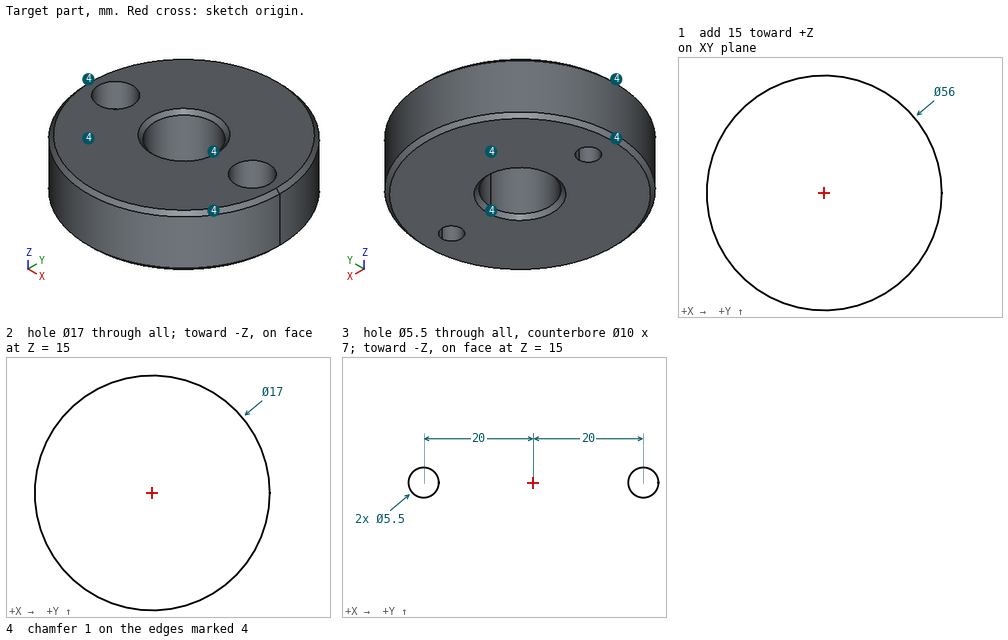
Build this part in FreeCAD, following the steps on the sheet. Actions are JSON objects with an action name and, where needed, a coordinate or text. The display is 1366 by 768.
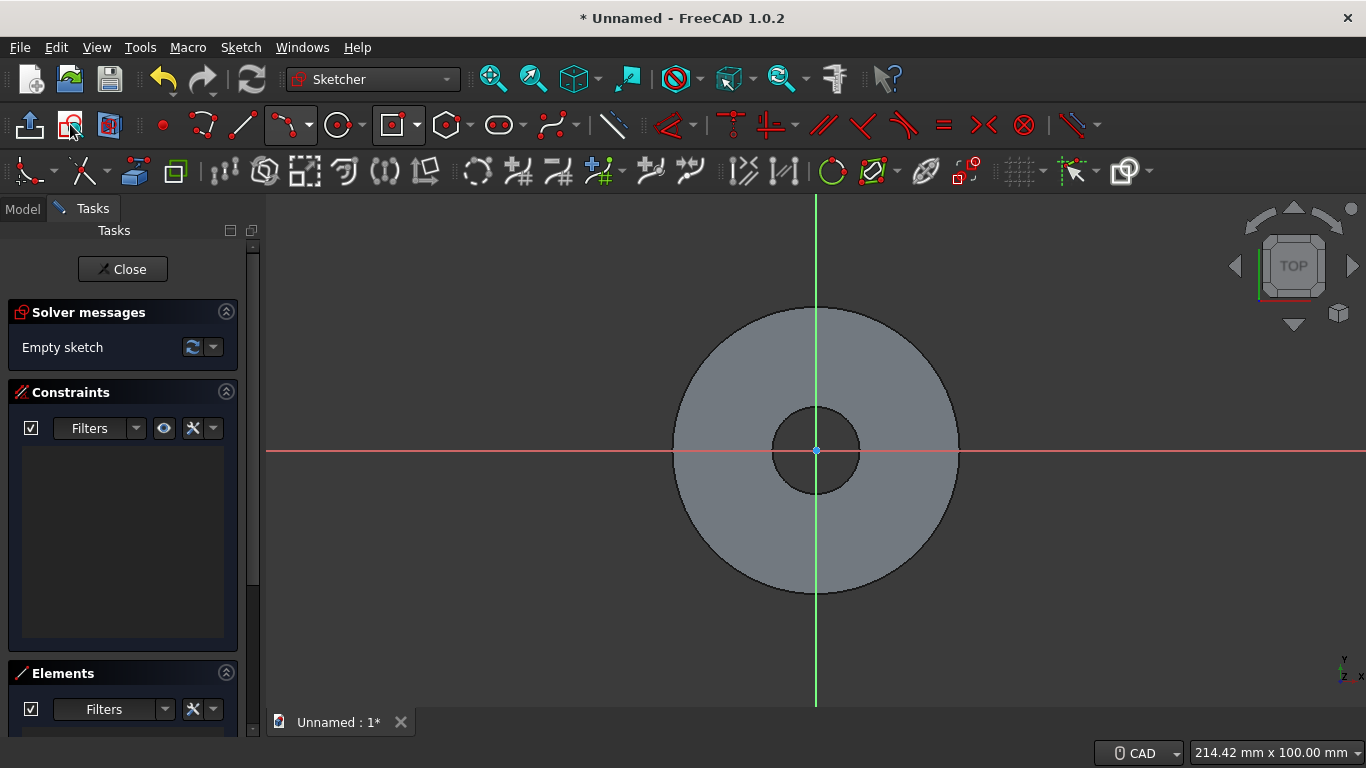
{"action": "scroll", "coordinate": [856, 450], "scroll_direction": "up", "scroll_amount": 5}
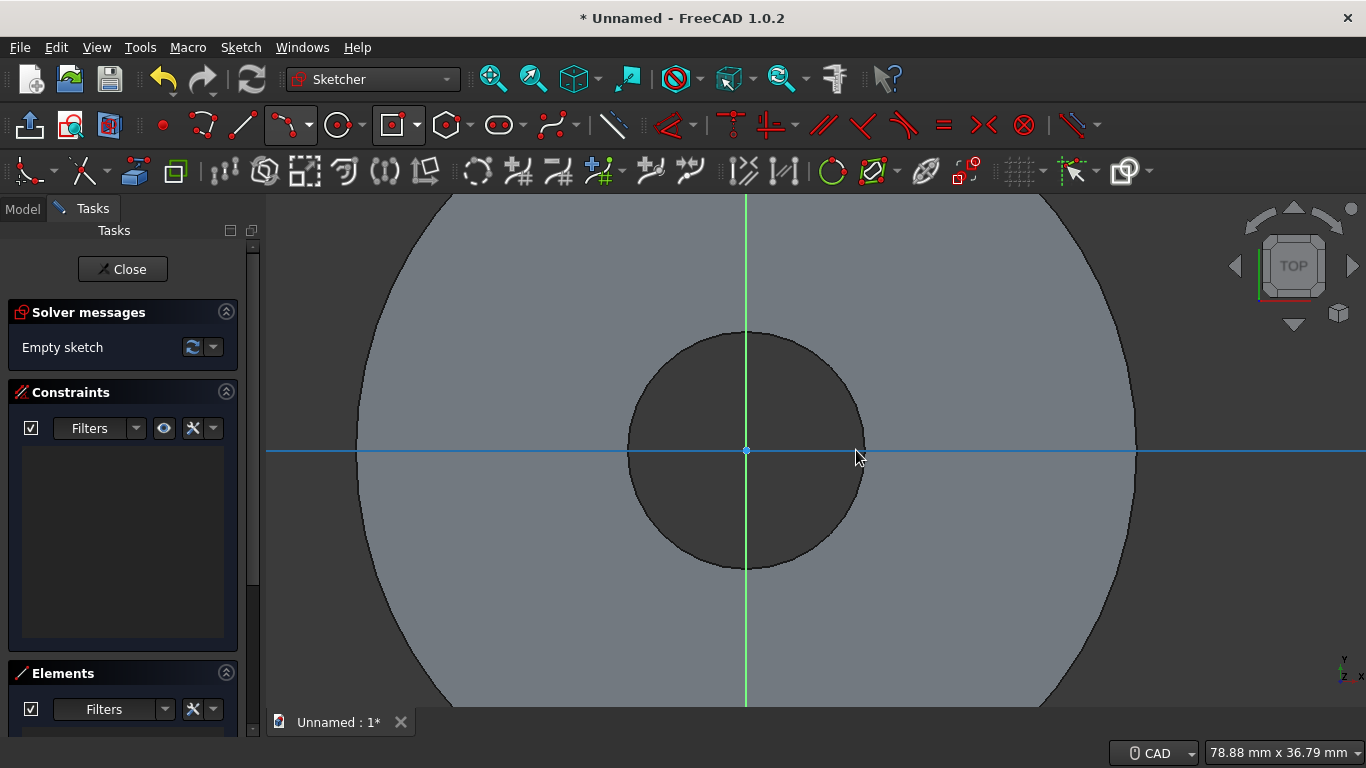
{"action": "left_click", "coordinate": [338, 126]}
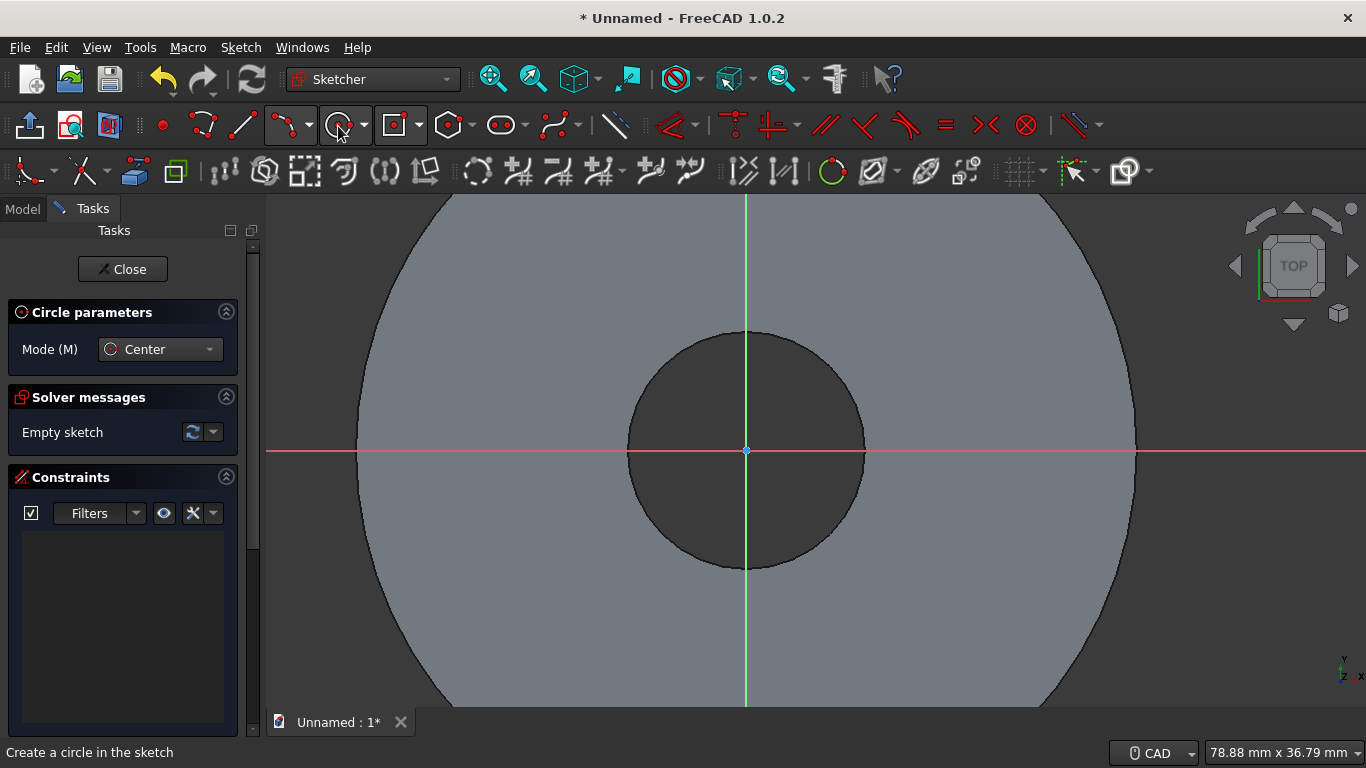
{"action": "left_click", "coordinate": [467, 450]}
{"action": "left_click", "coordinate": [495, 423]}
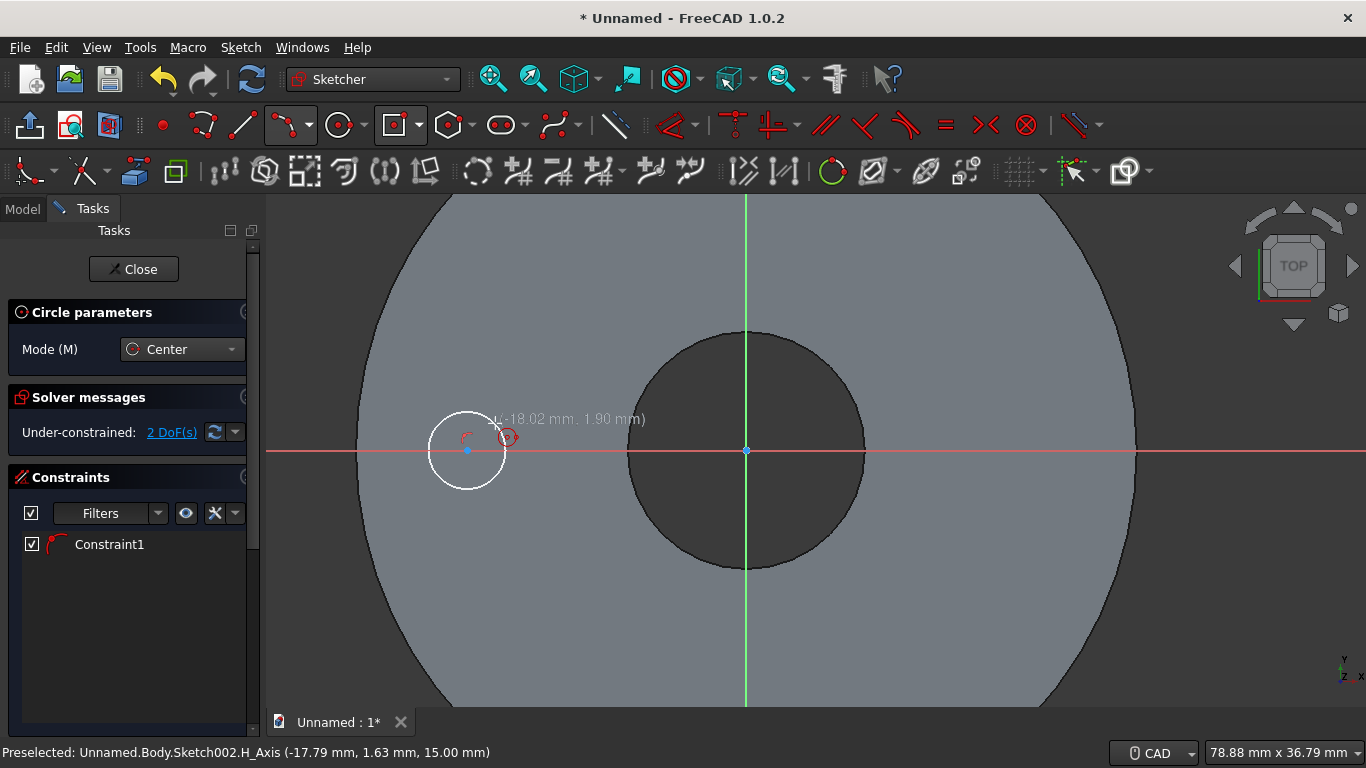
{"action": "left_click", "coordinate": [1025, 450]}
{"action": "left_click", "coordinate": [1052, 423]}
{"action": "key", "text": "Escape"}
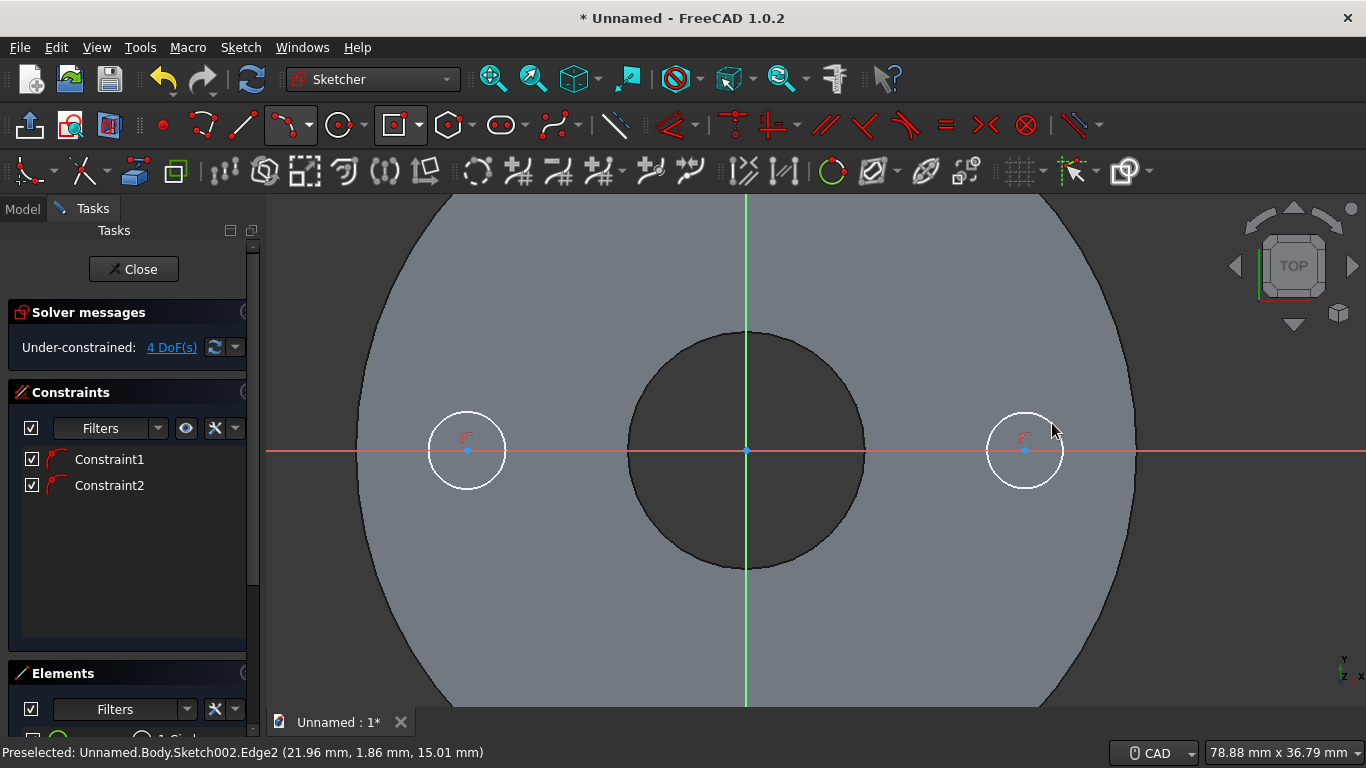
{"action": "left_click", "coordinate": [494, 423]}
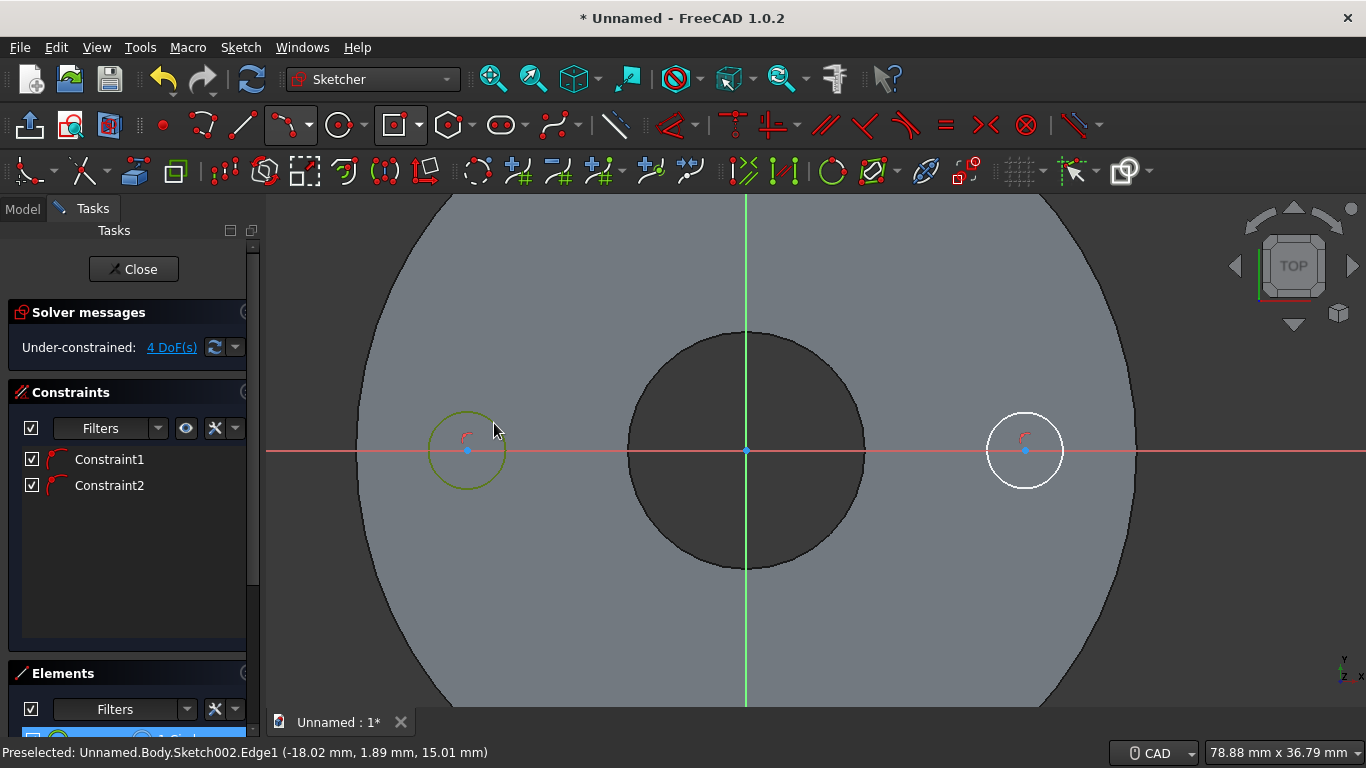
{"action": "left_click", "coordinate": [1052, 424]}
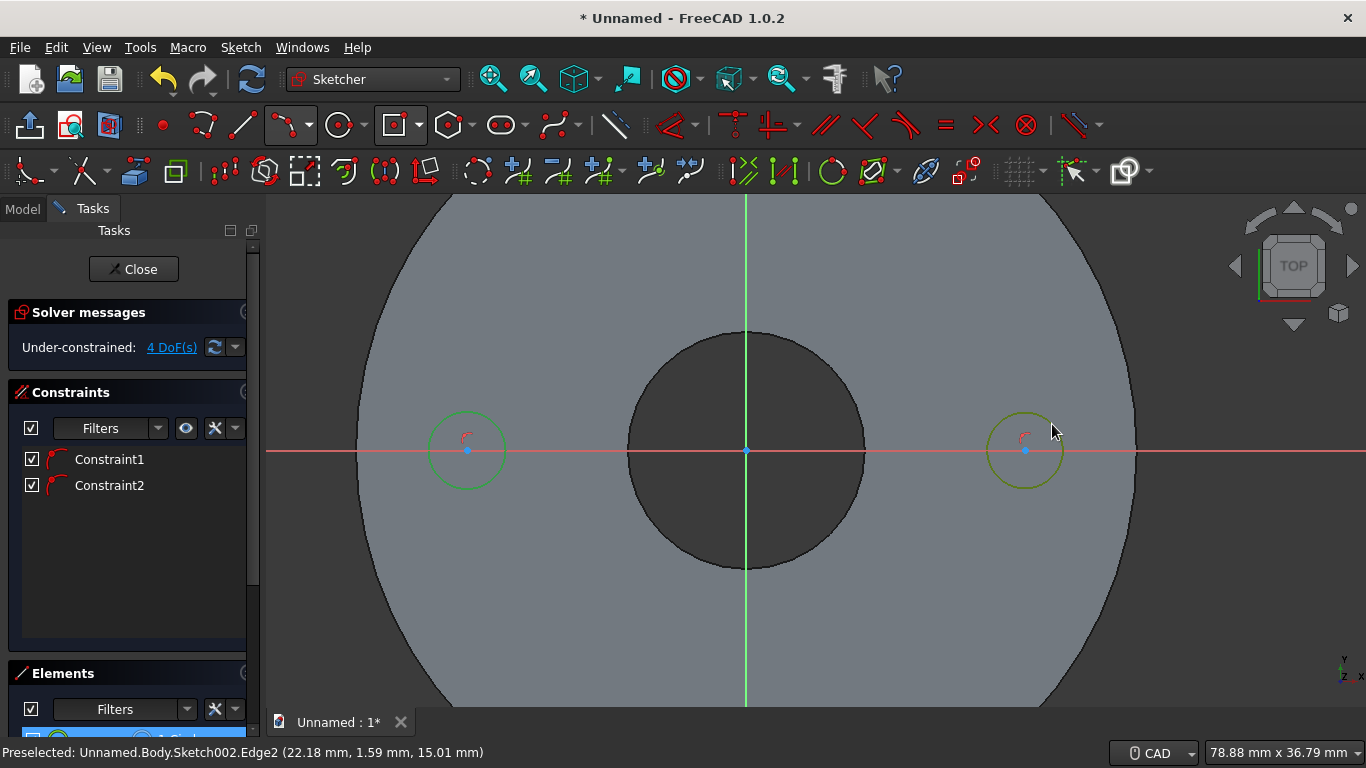
{"action": "left_click", "coordinate": [946, 126]}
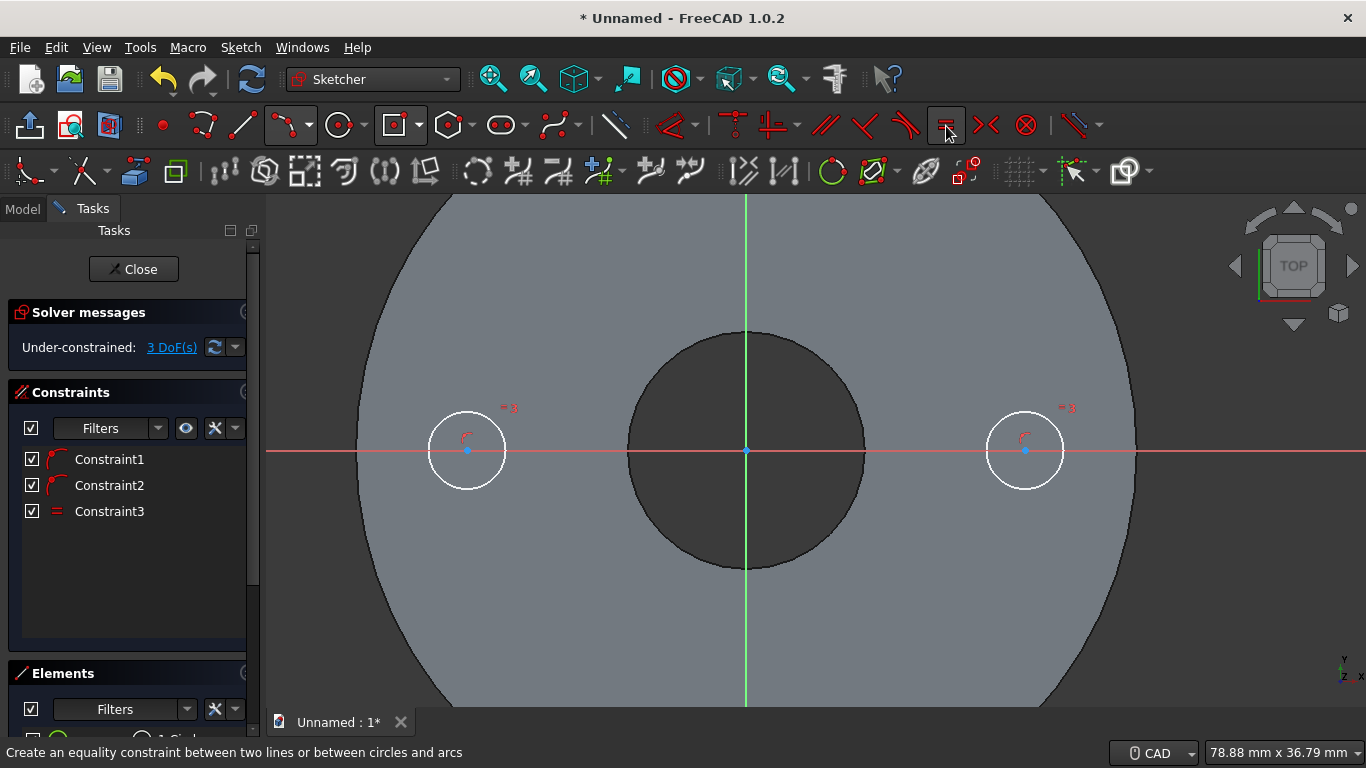
{"action": "left_click", "coordinate": [670, 126]}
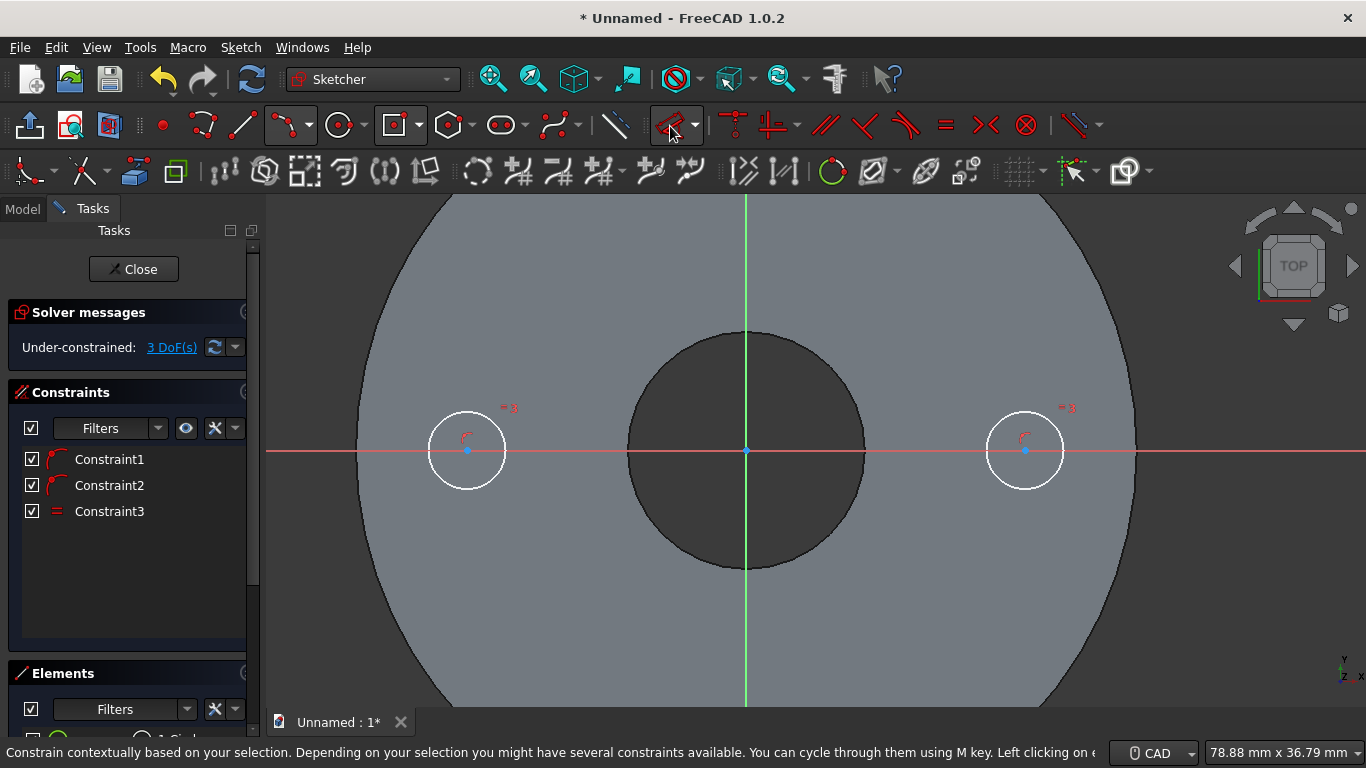
{"action": "left_click", "coordinate": [494, 423]}
{"action": "left_click", "coordinate": [516, 400]}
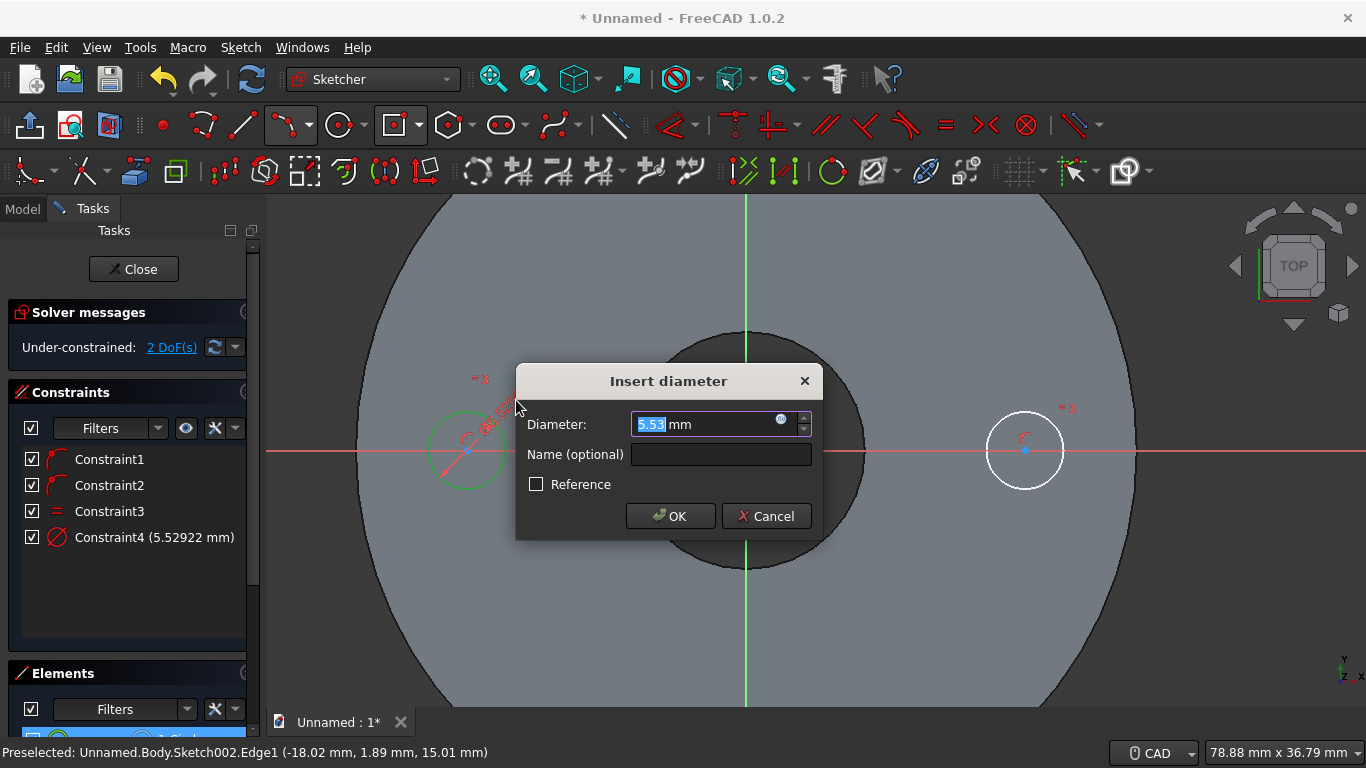
{"action": "type", "text": "5.5"}
{"action": "key", "text": "Return"}